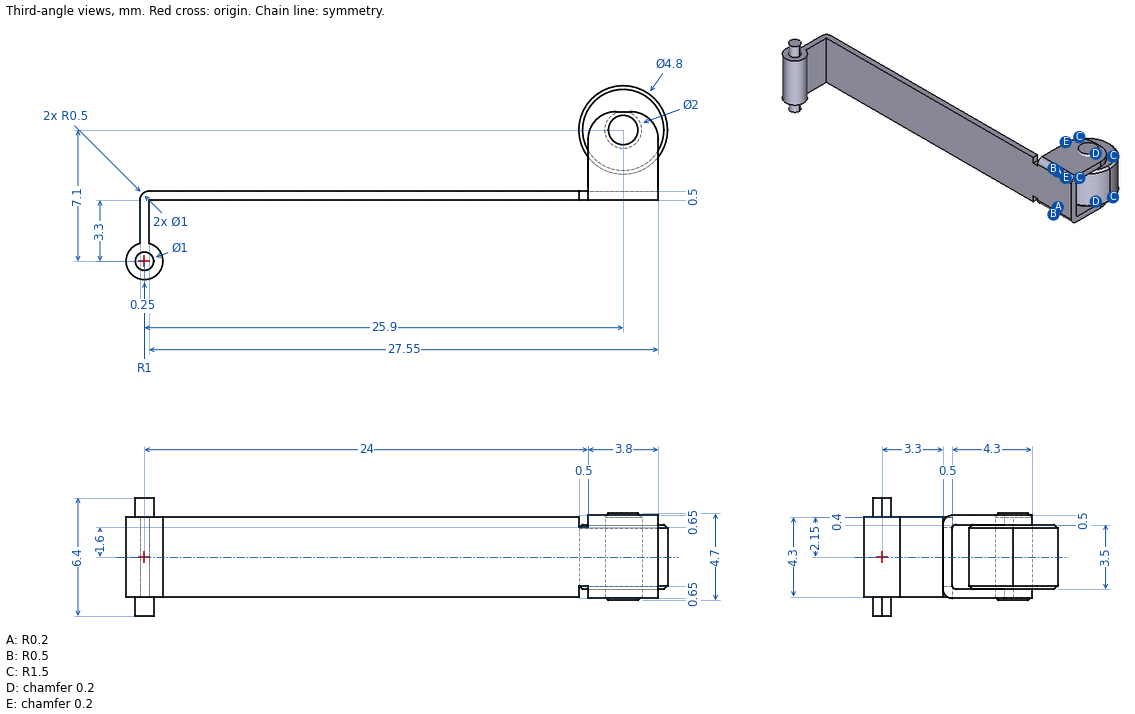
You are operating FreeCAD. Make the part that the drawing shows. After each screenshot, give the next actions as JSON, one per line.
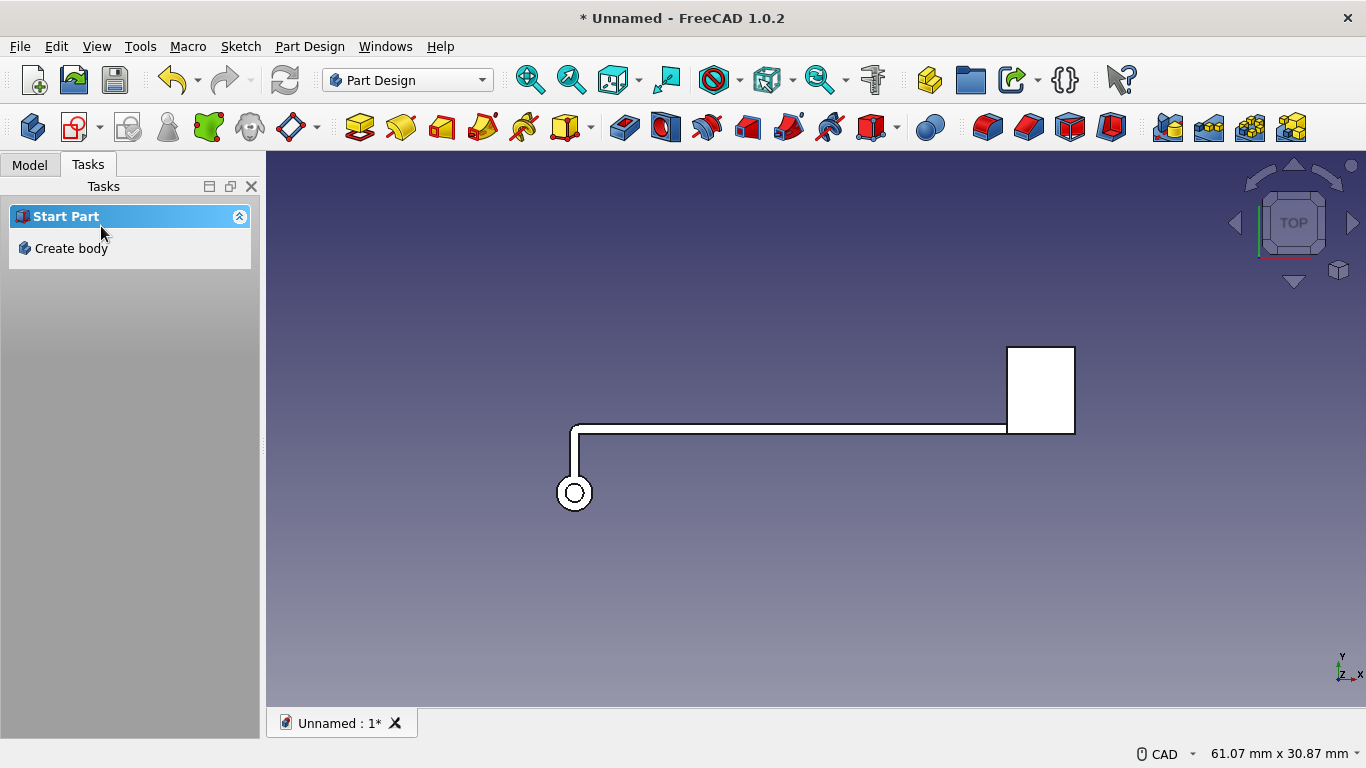
{"action": "key", "text": "4"}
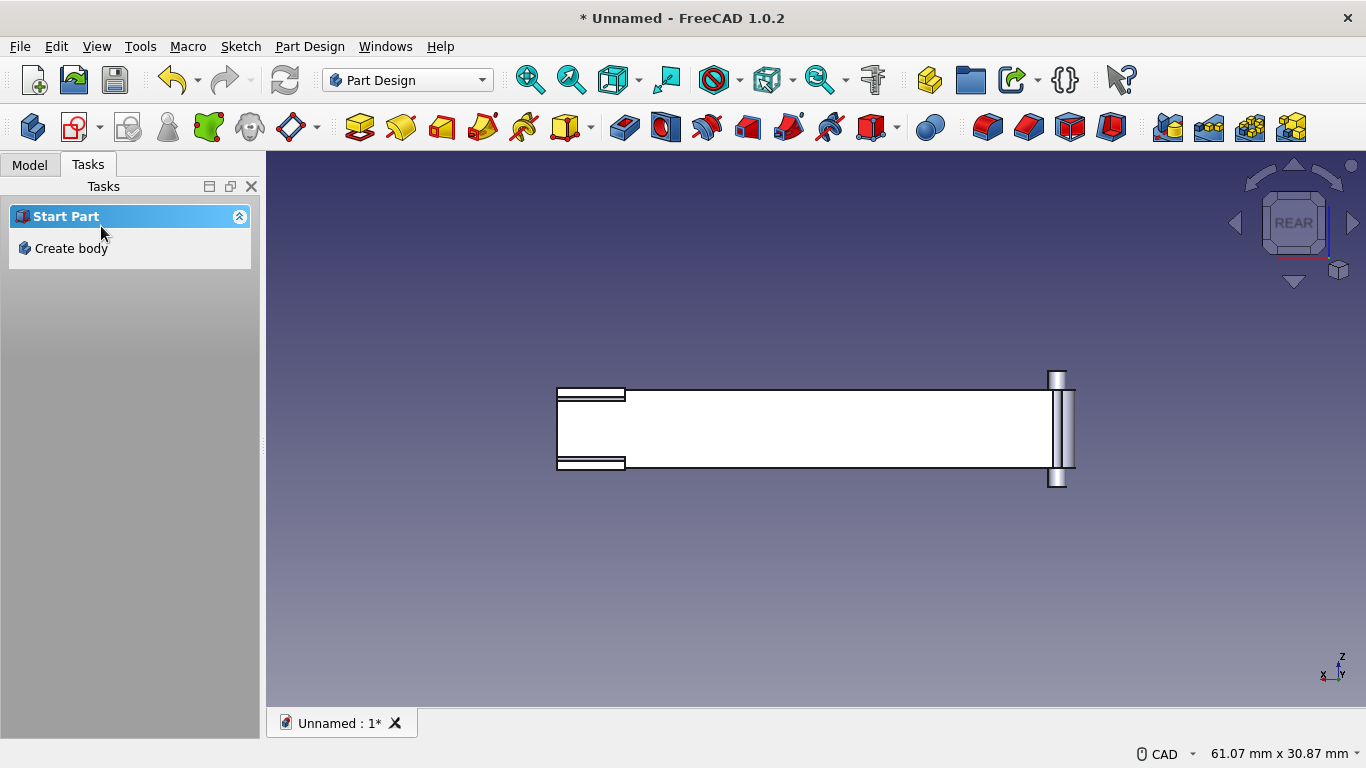
{"action": "left_click", "coordinate": [663, 428]}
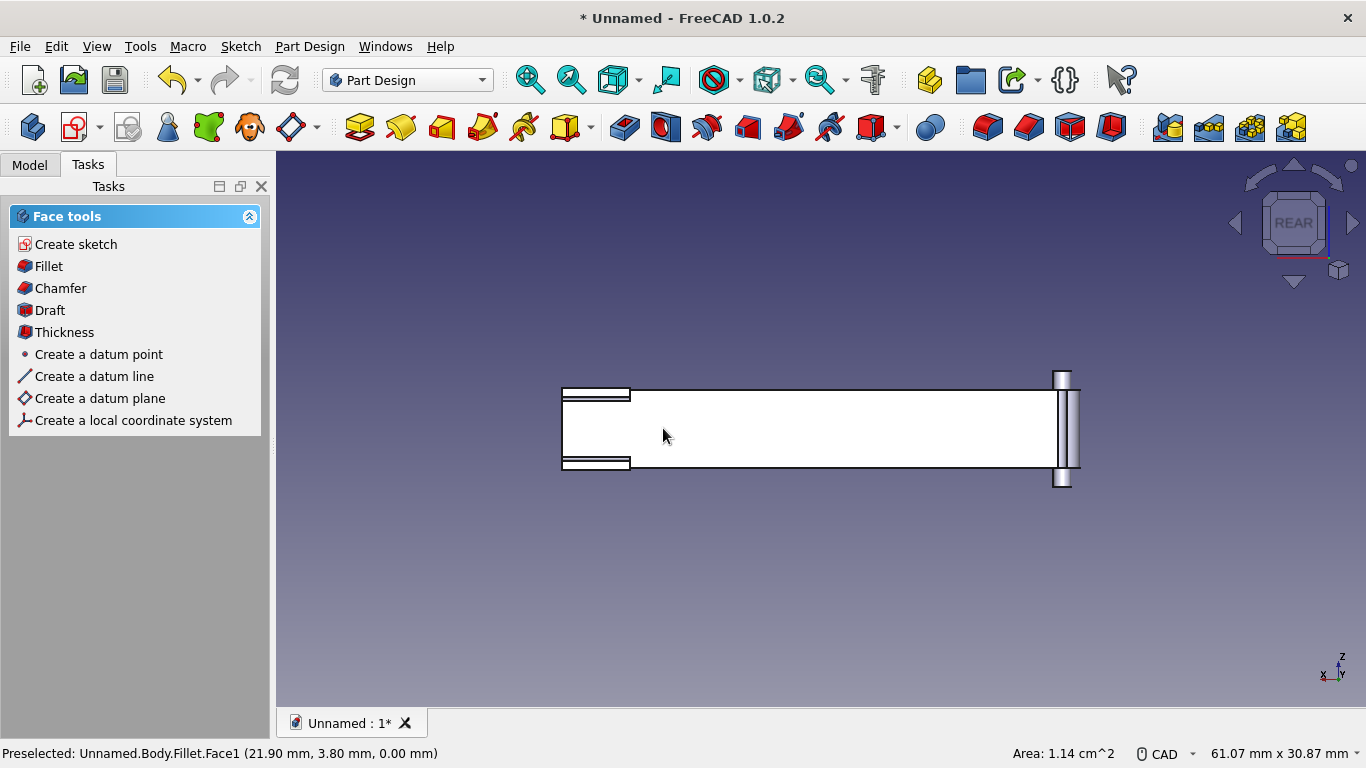
{"action": "left_click", "coordinate": [74, 128]}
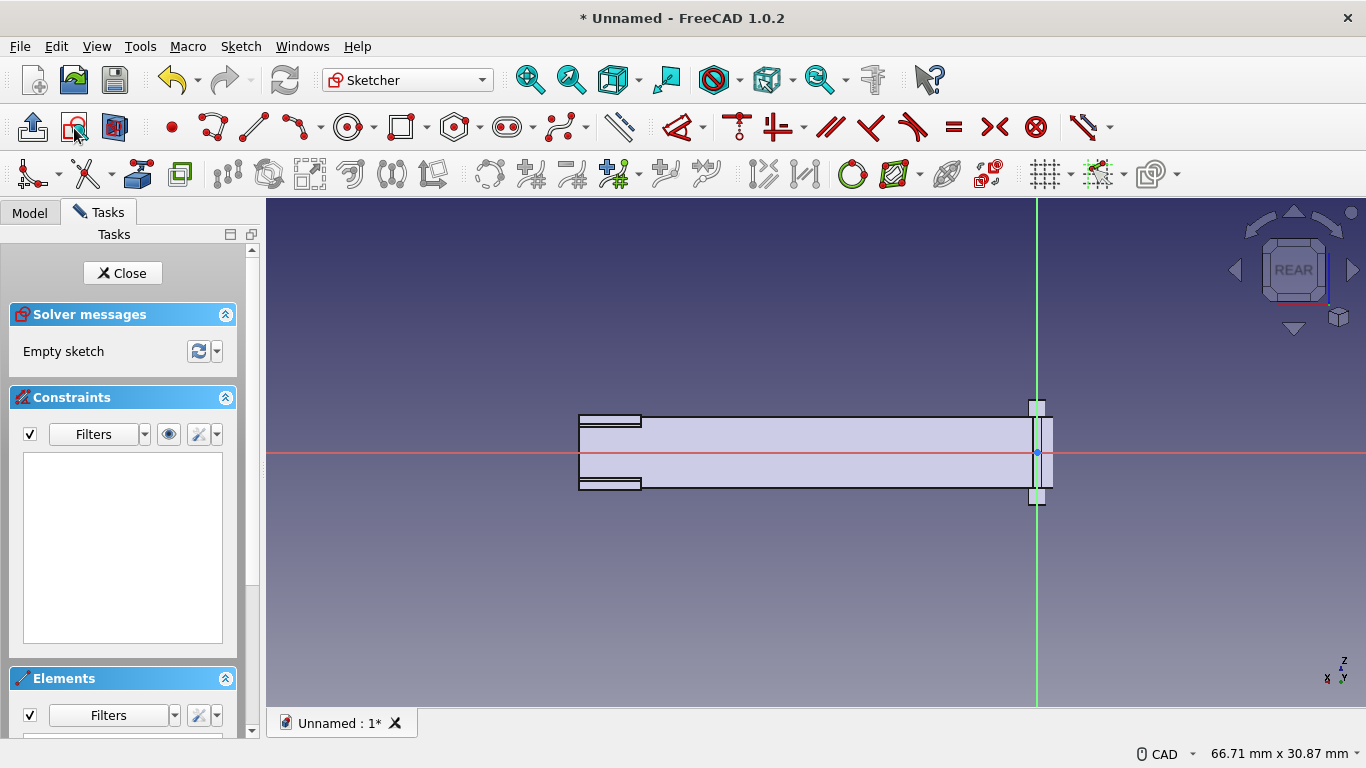
{"action": "left_click", "coordinate": [115, 128]}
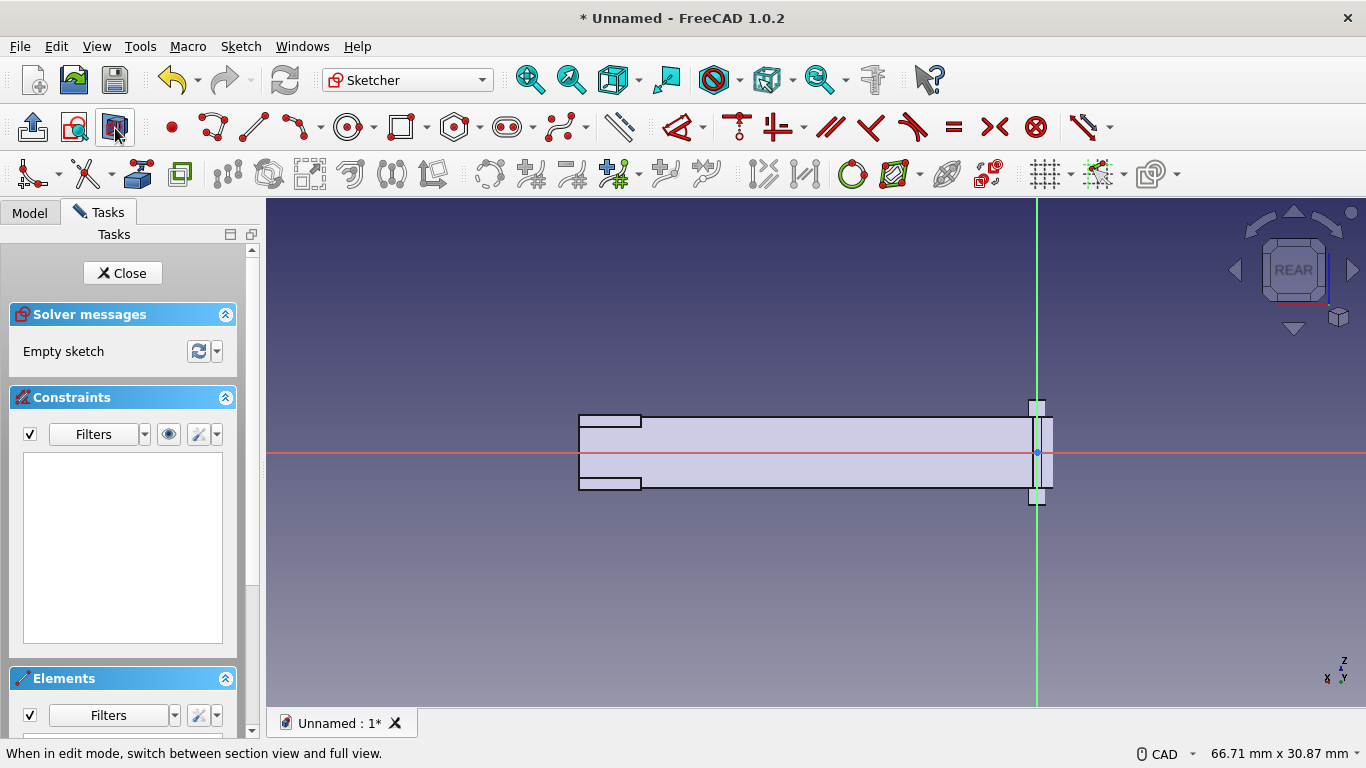
{"action": "scroll", "coordinate": [612, 453], "scroll_direction": "up", "scroll_amount": 7}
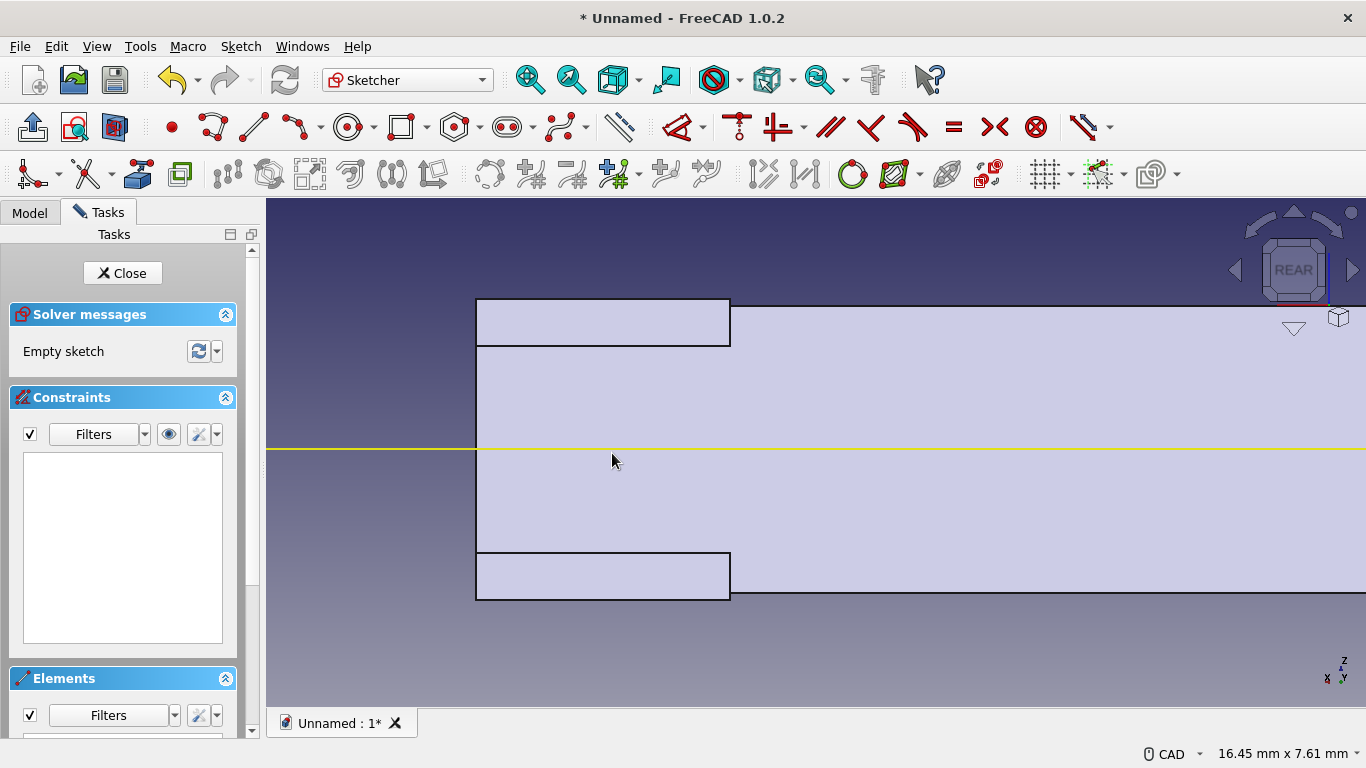
{"action": "key", "text": "g r"}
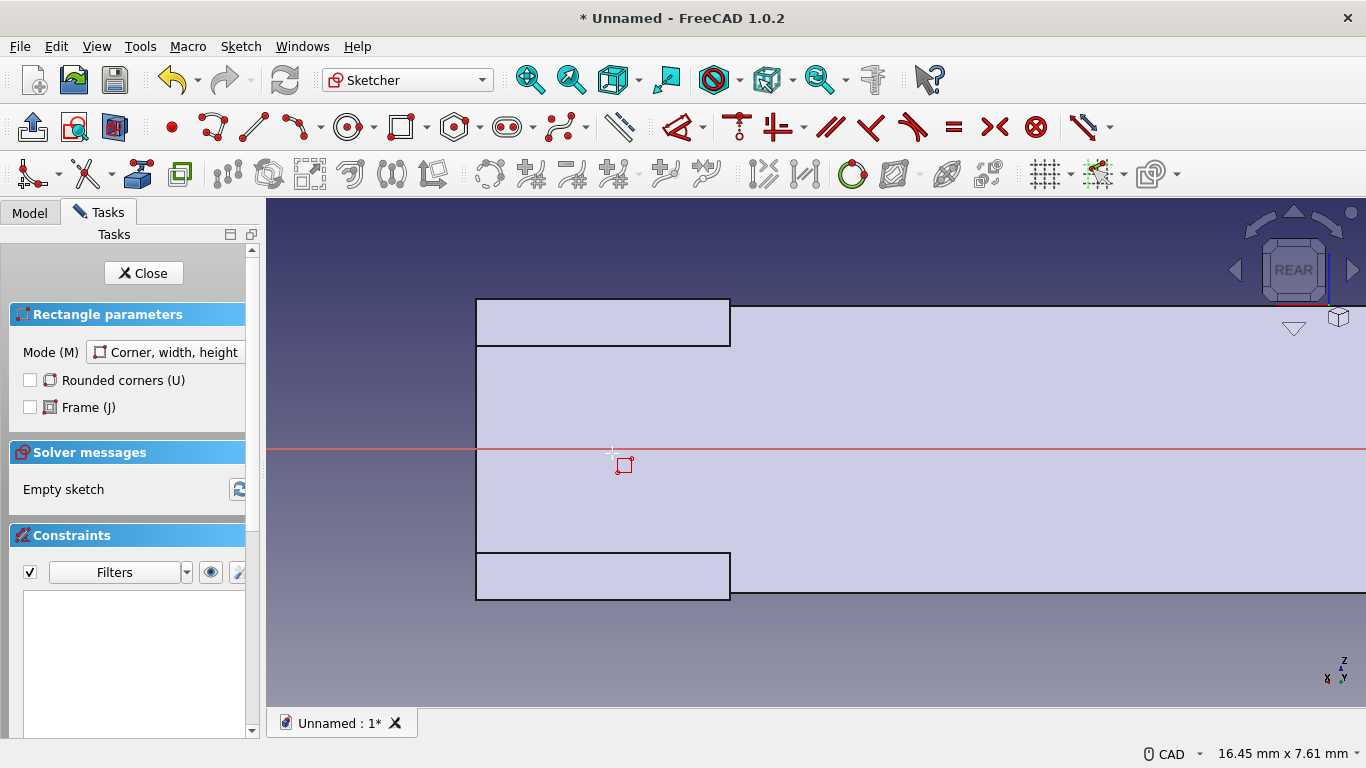
{"action": "left_click", "coordinate": [730, 299]}
{"action": "mouse_move", "coordinate": [763, 342]}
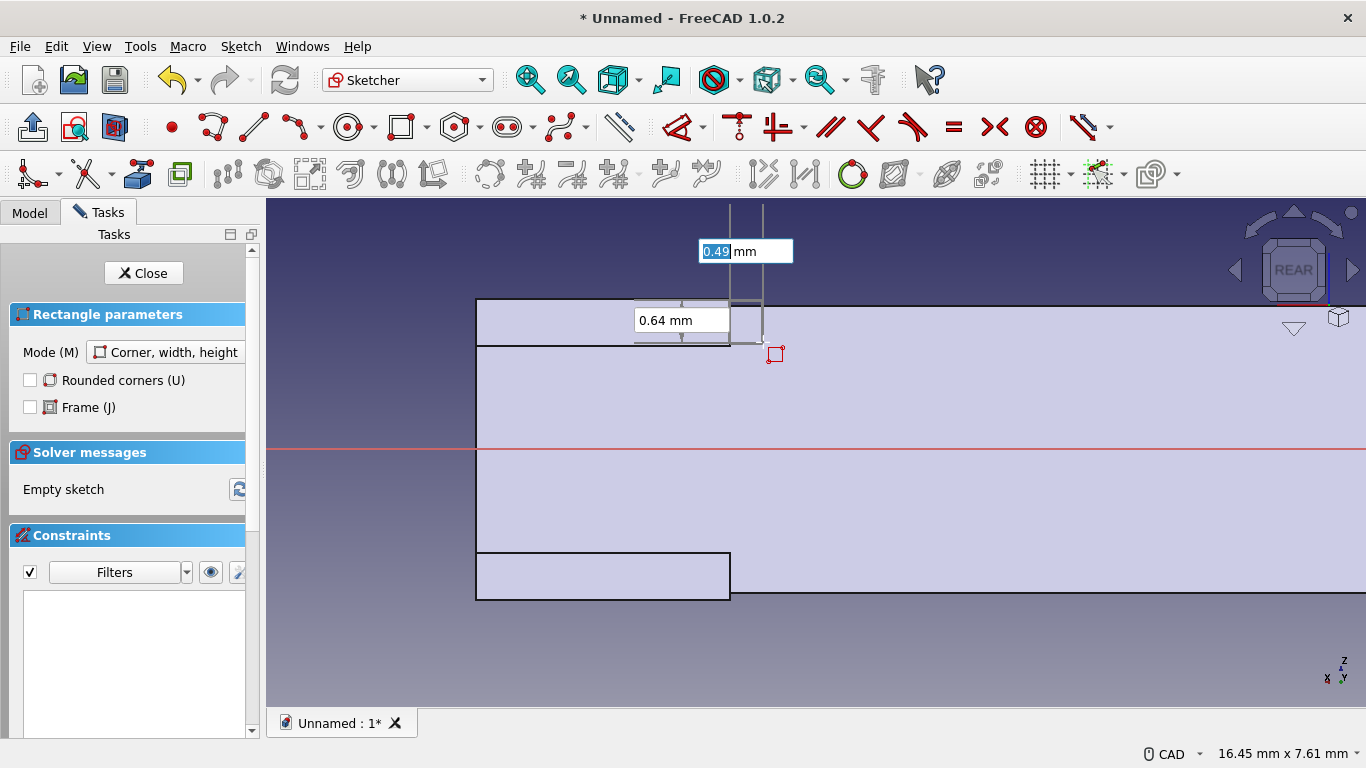
{"action": "type", "text": "0.5"}
{"action": "key", "text": "Tab"}
{"action": "type", "text": "0.65"}
{"action": "key", "text": "Return"}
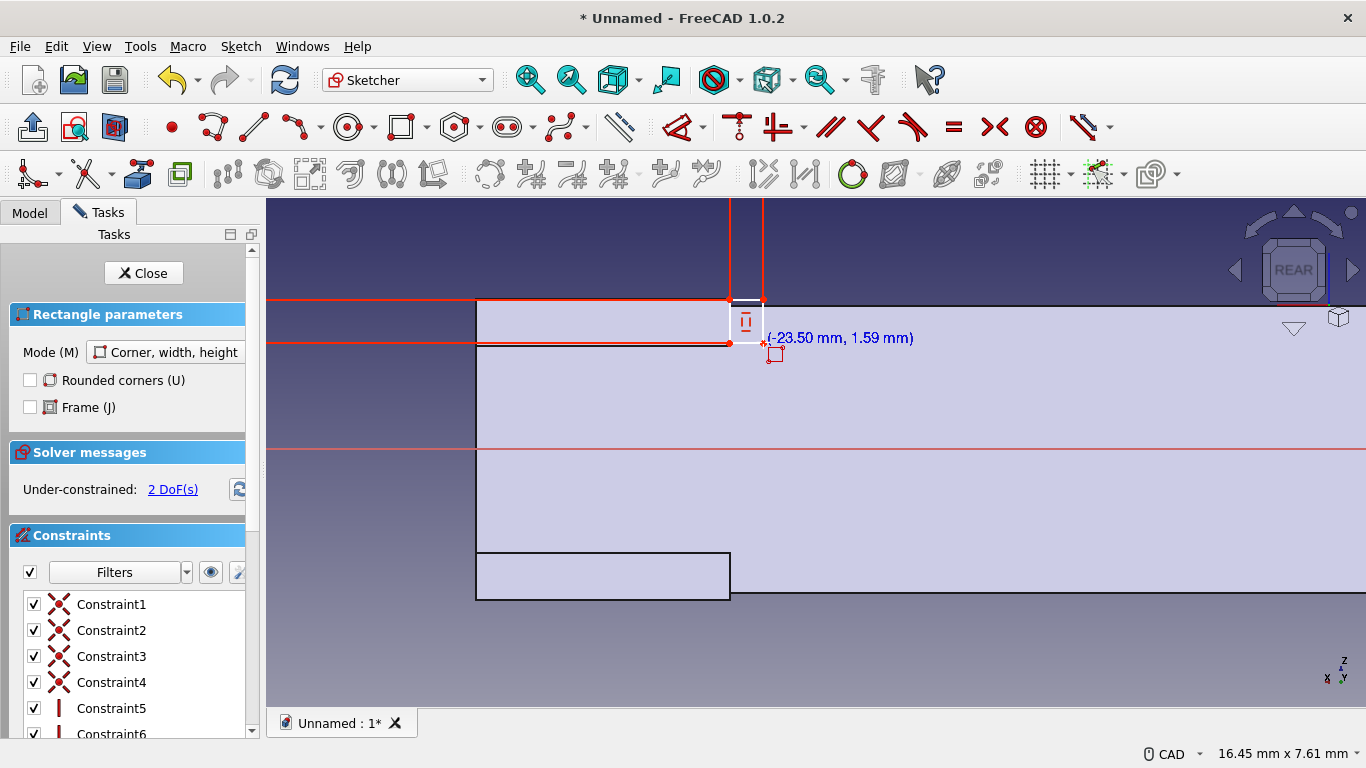
{"action": "left_click", "coordinate": [730, 556]}
{"action": "mouse_move", "coordinate": [763, 600]}